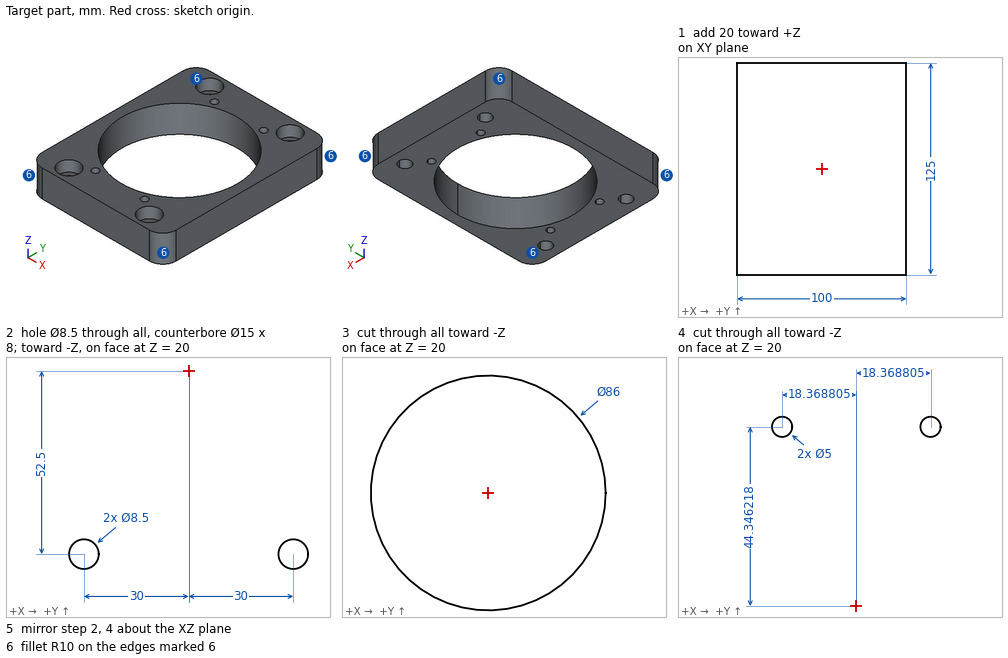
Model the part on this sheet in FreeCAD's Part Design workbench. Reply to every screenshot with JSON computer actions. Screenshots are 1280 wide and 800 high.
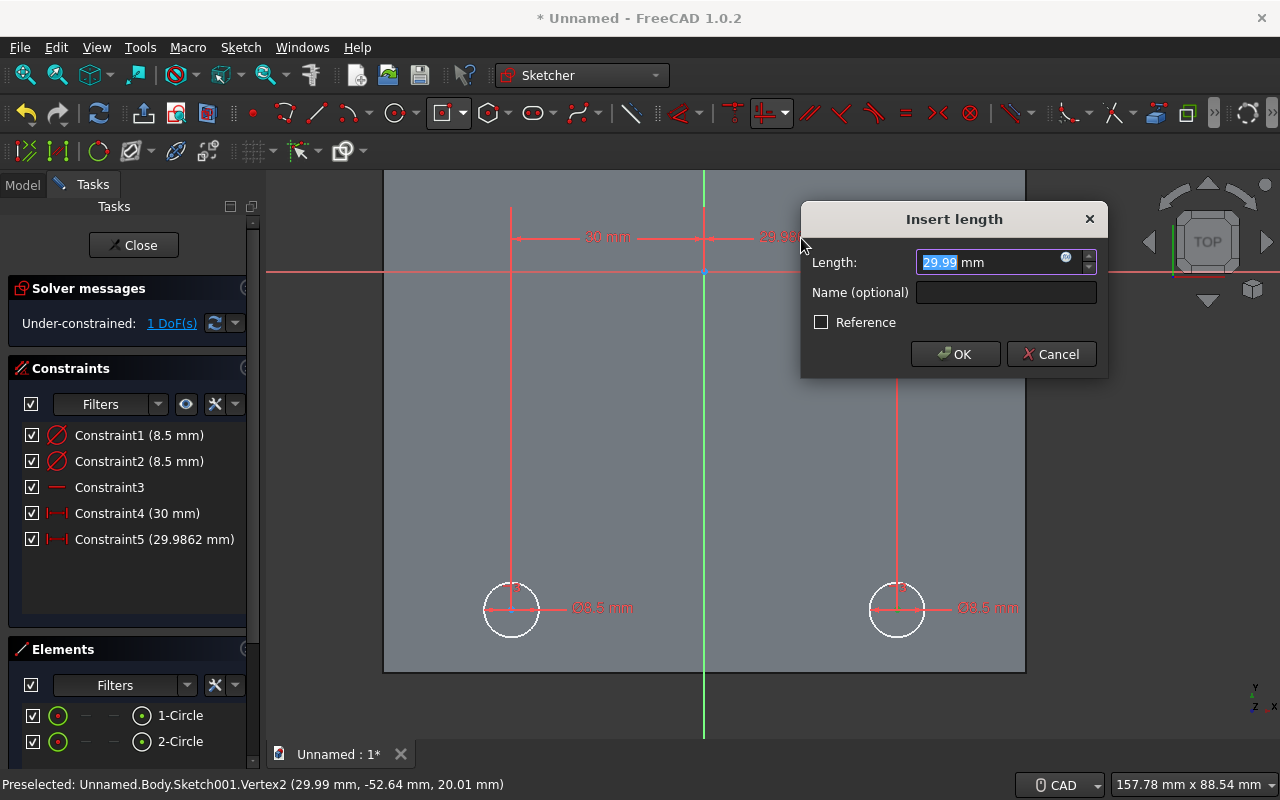
{"action": "type", "text": "30"}
{"action": "key", "text": "Return"}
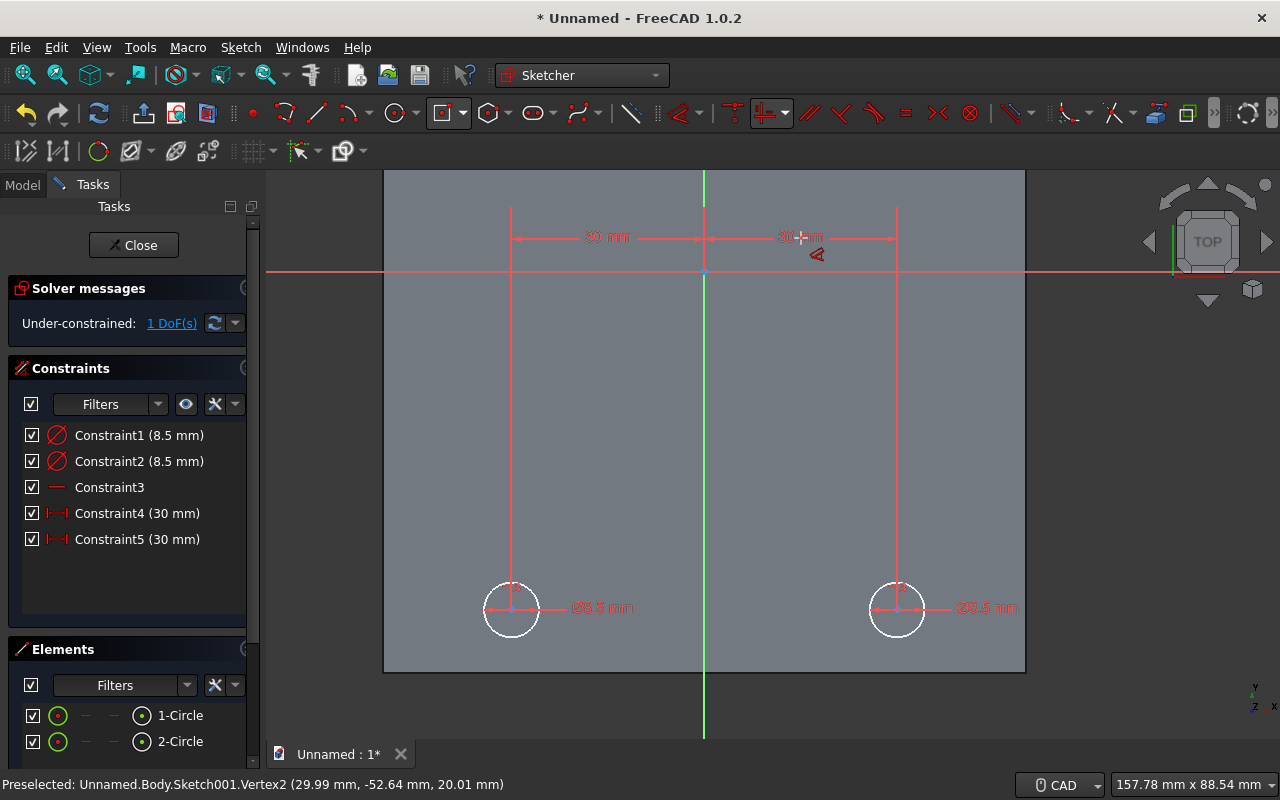
{"action": "left_click", "coordinate": [511, 610]}
{"action": "left_click", "coordinate": [477, 441]}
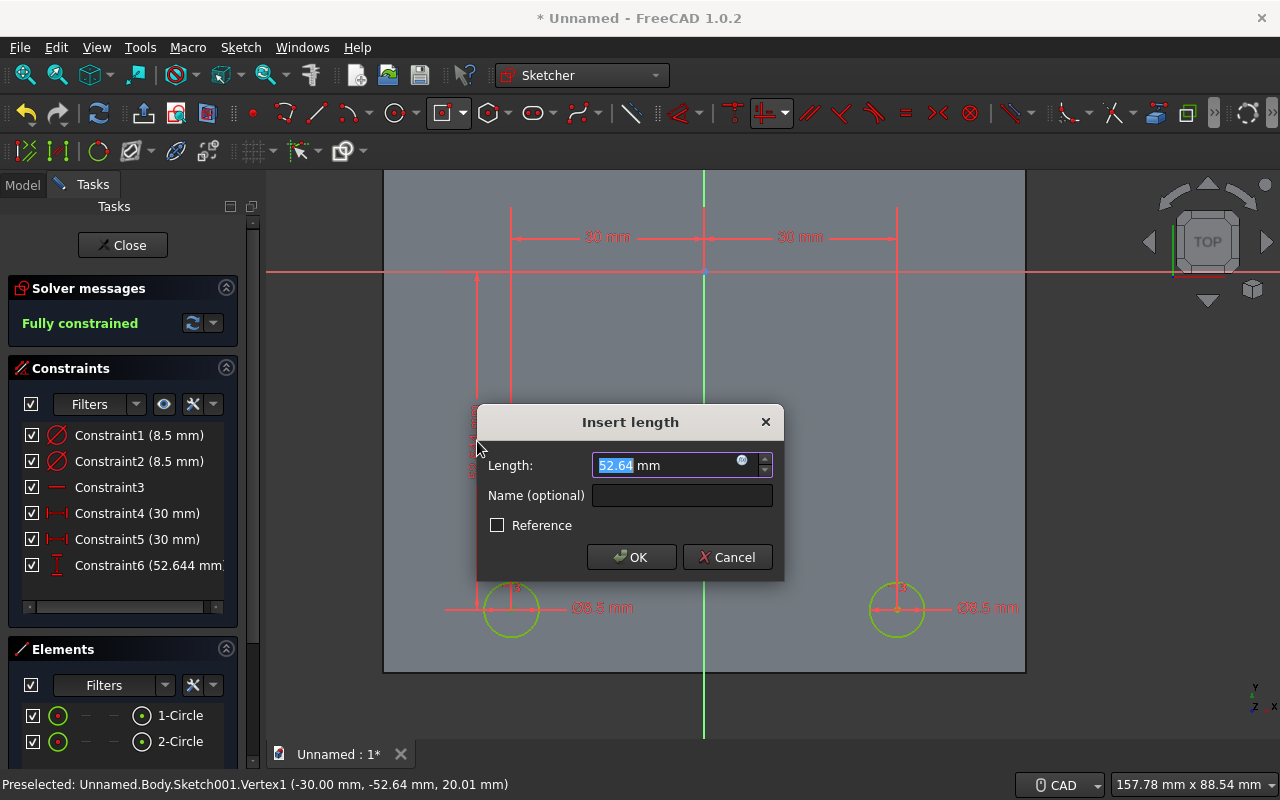
{"action": "type", "text": "52.5"}
{"action": "key", "text": "Return"}
{"action": "key", "text": "Escape"}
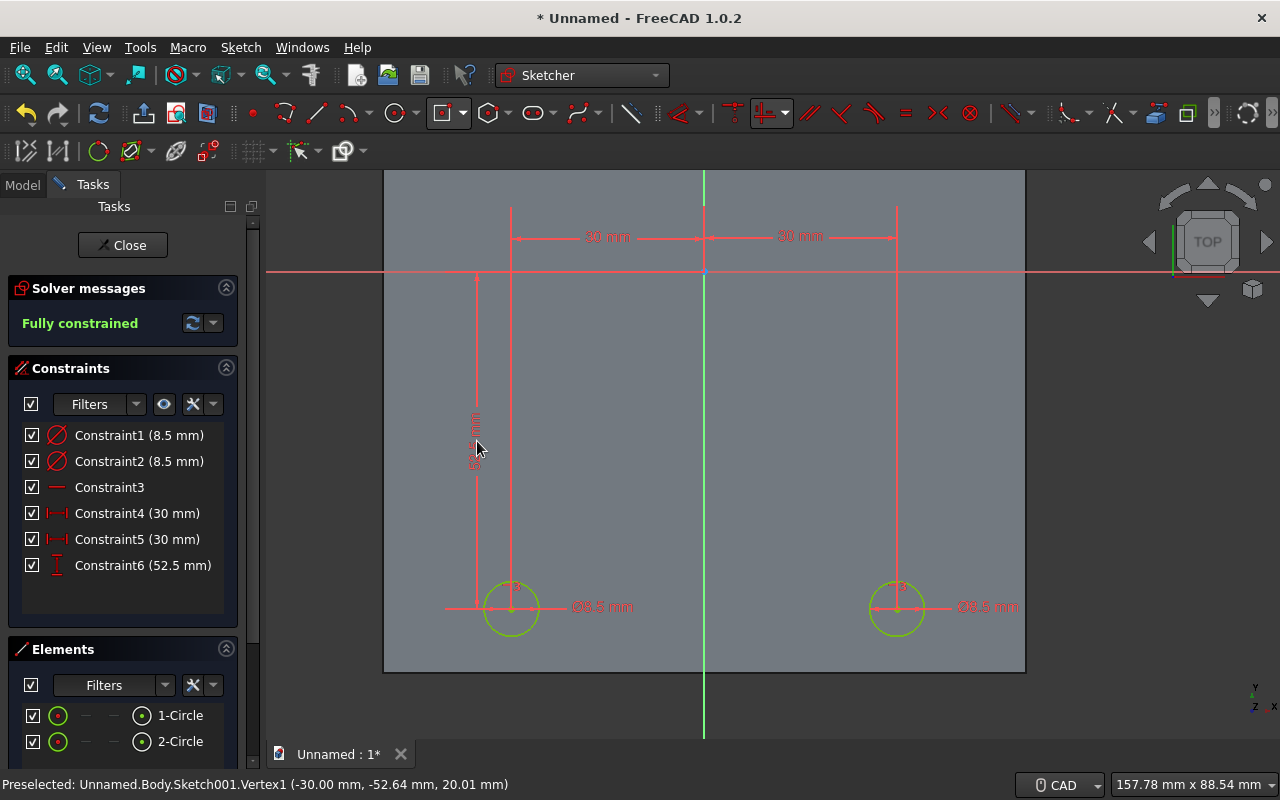
{"action": "left_click", "coordinate": [123, 245]}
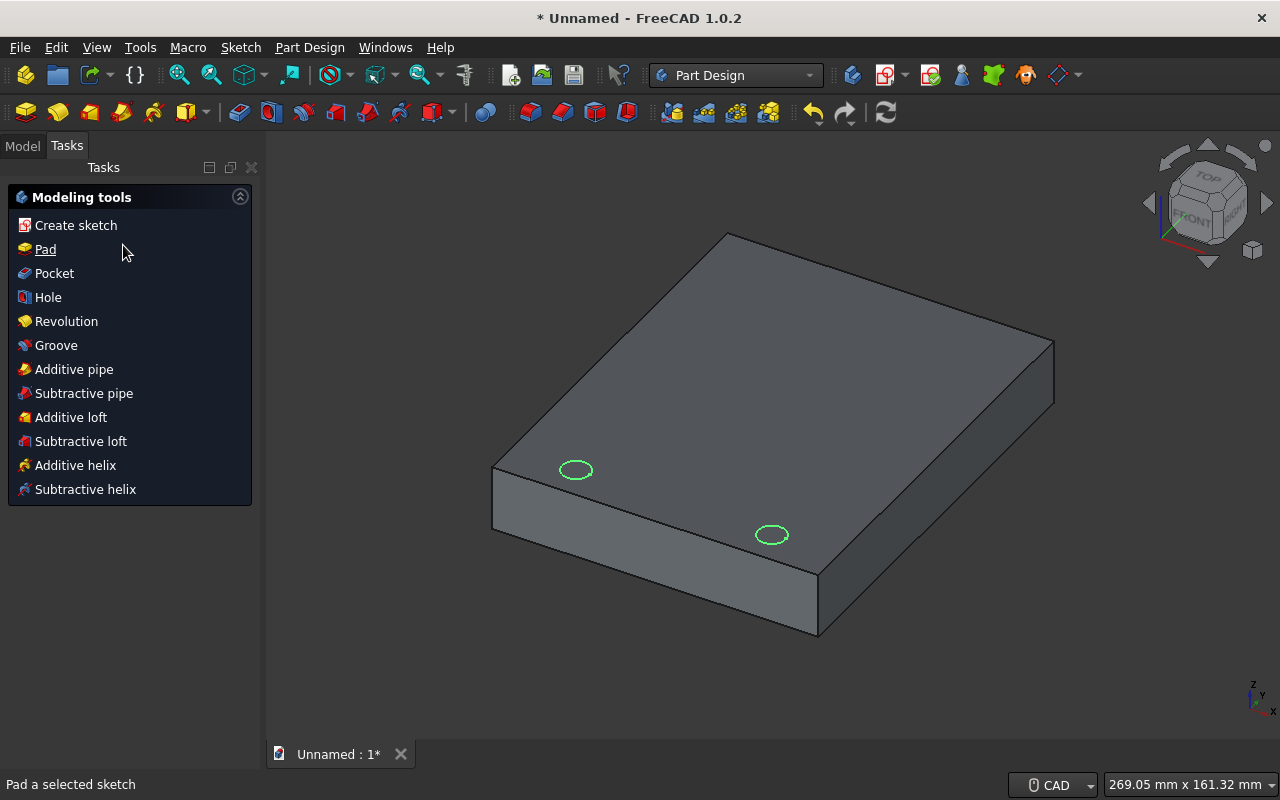
{"action": "left_click", "coordinate": [272, 112]}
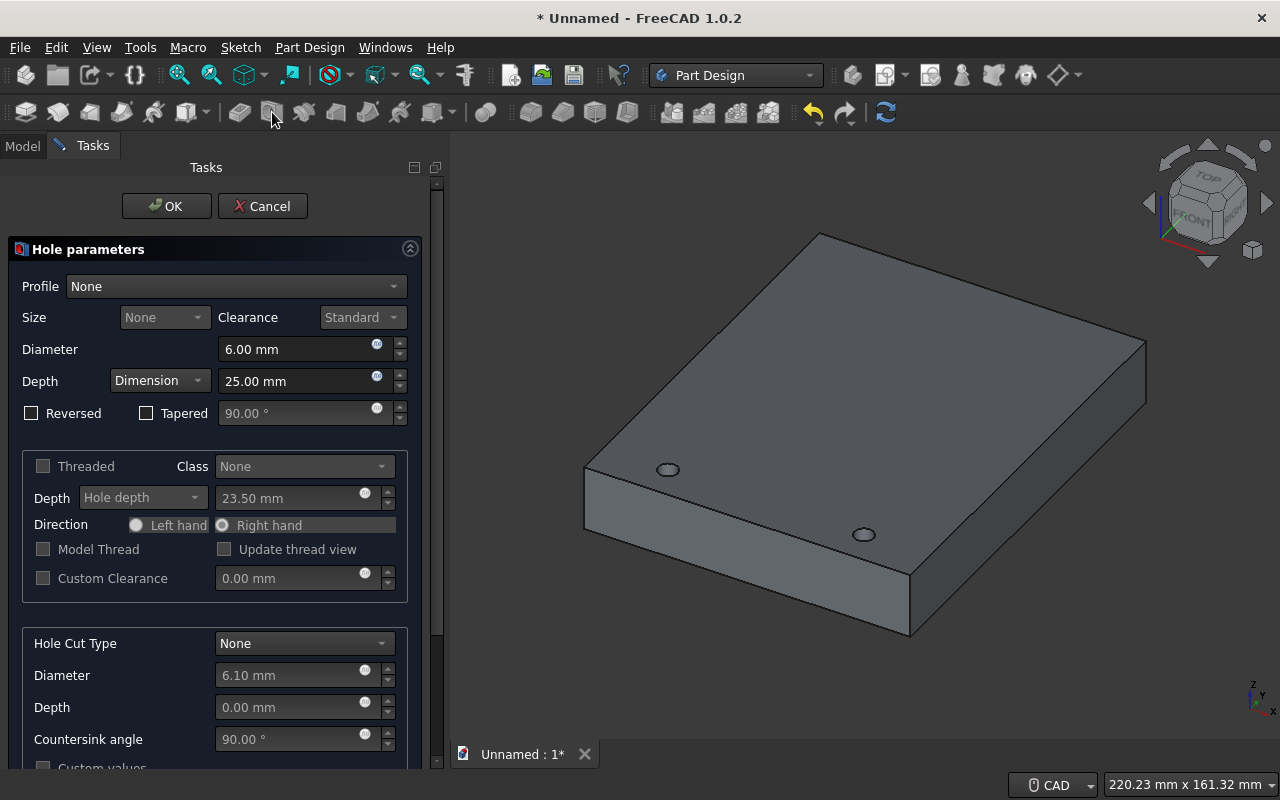
{"action": "triple_click", "coordinate": [305, 349]}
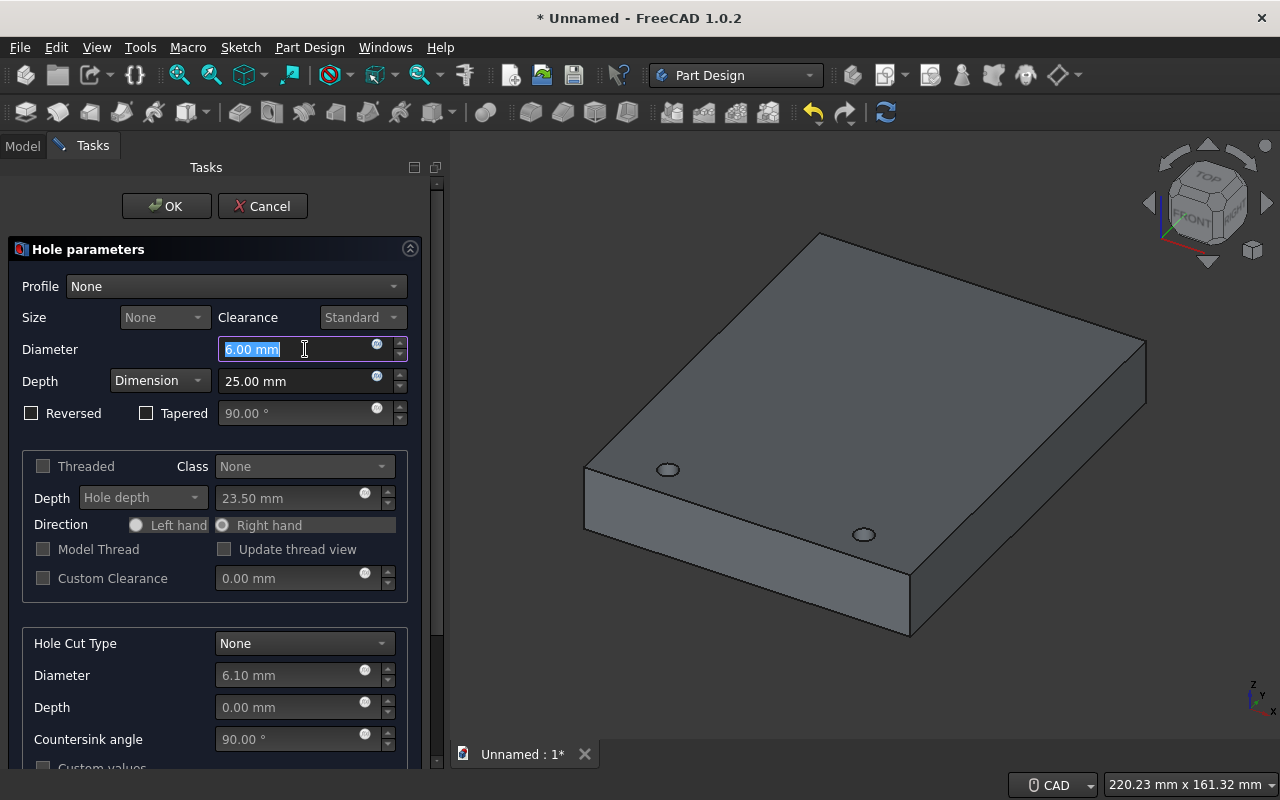
{"action": "type", "text": "8.5"}
{"action": "key", "text": "Tab"}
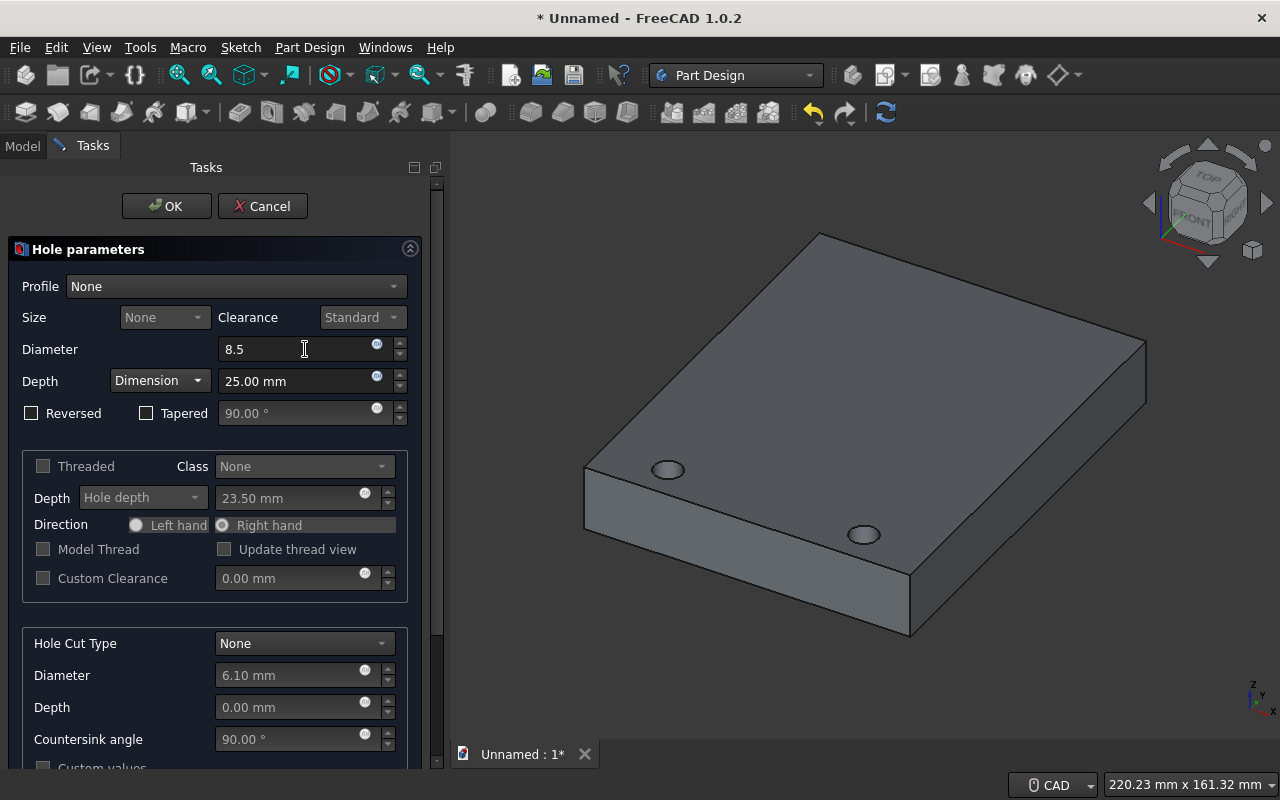
{"action": "left_click", "coordinate": [161, 380]}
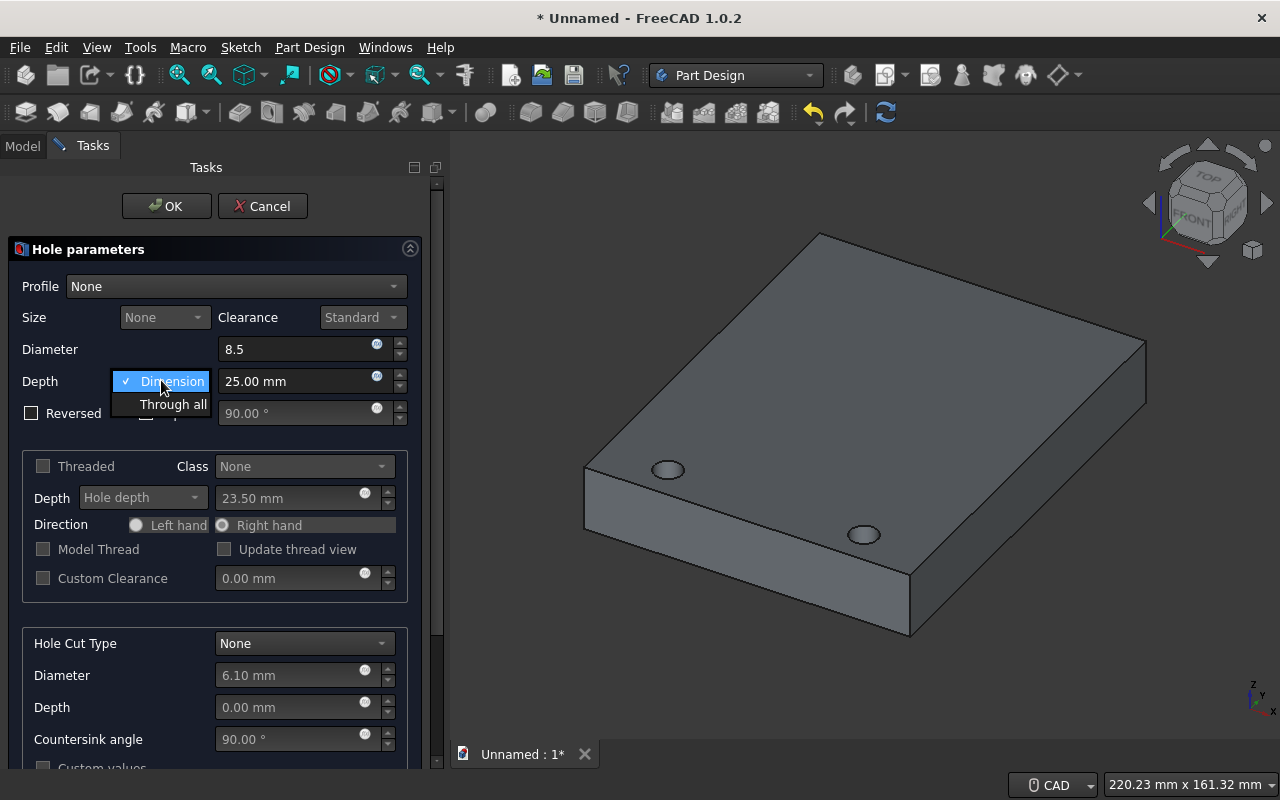
{"action": "left_click", "coordinate": [160, 404]}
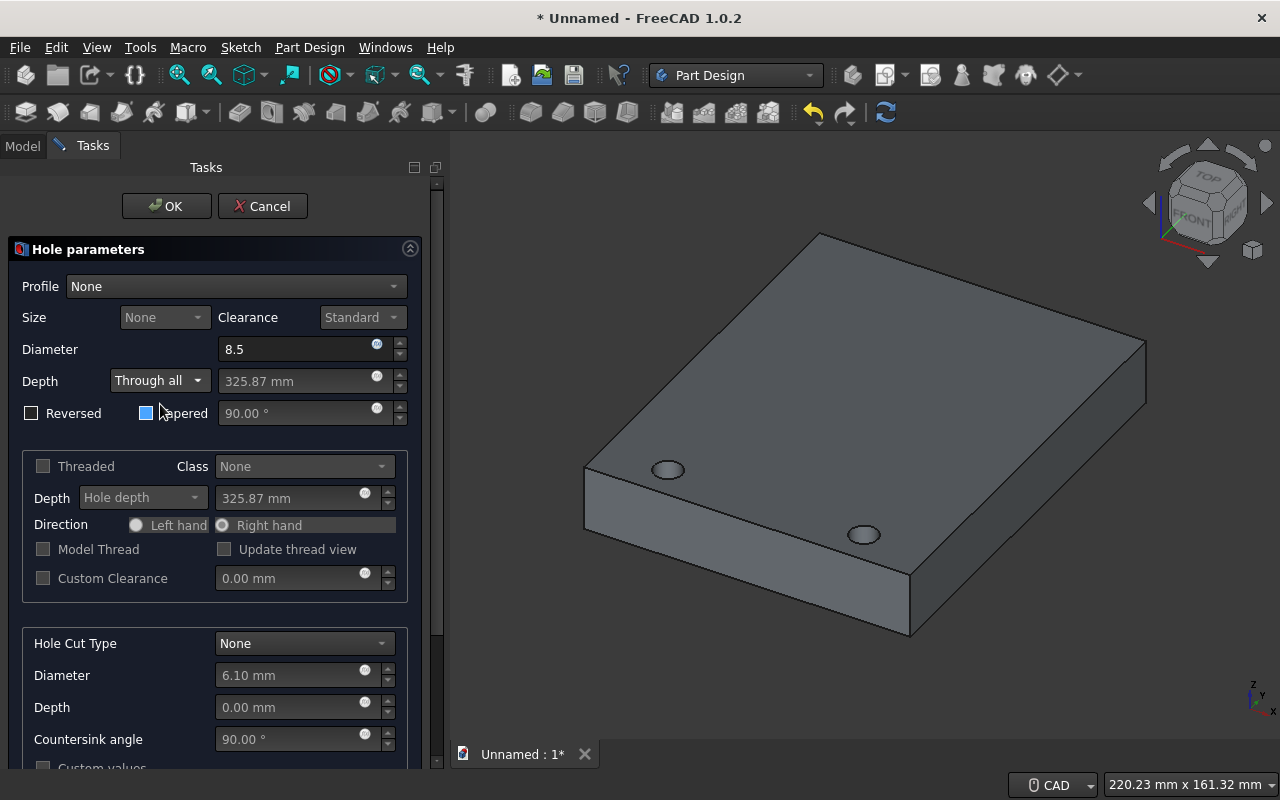
{"action": "left_click", "coordinate": [306, 644]}